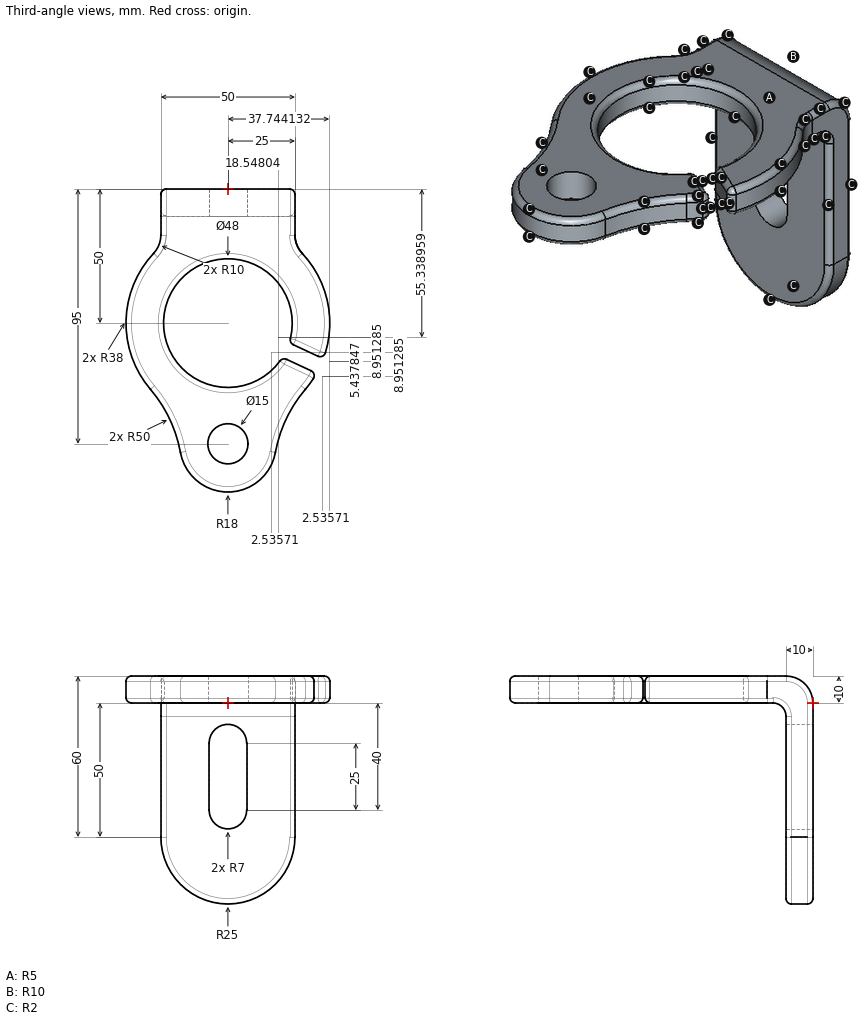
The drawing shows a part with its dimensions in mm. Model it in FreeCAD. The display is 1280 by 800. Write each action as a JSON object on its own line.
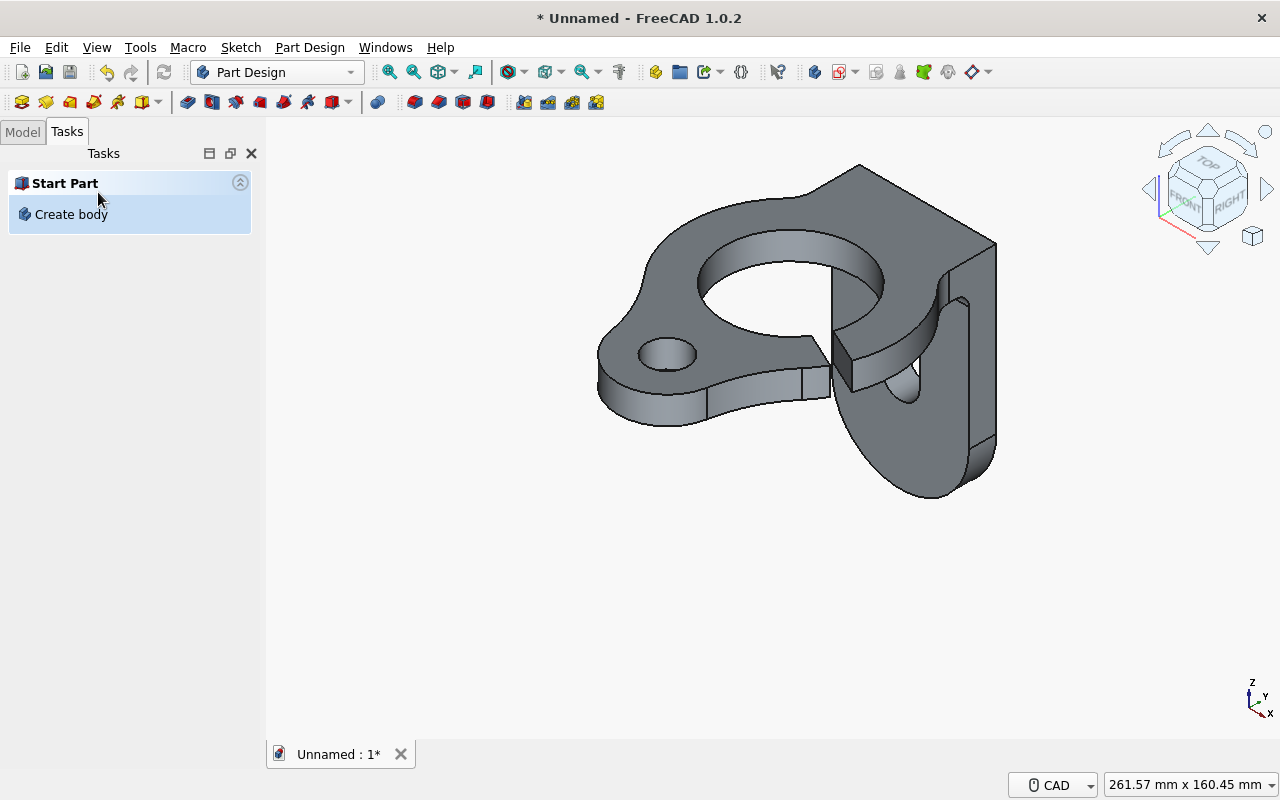
{"action": "key", "text": "2"}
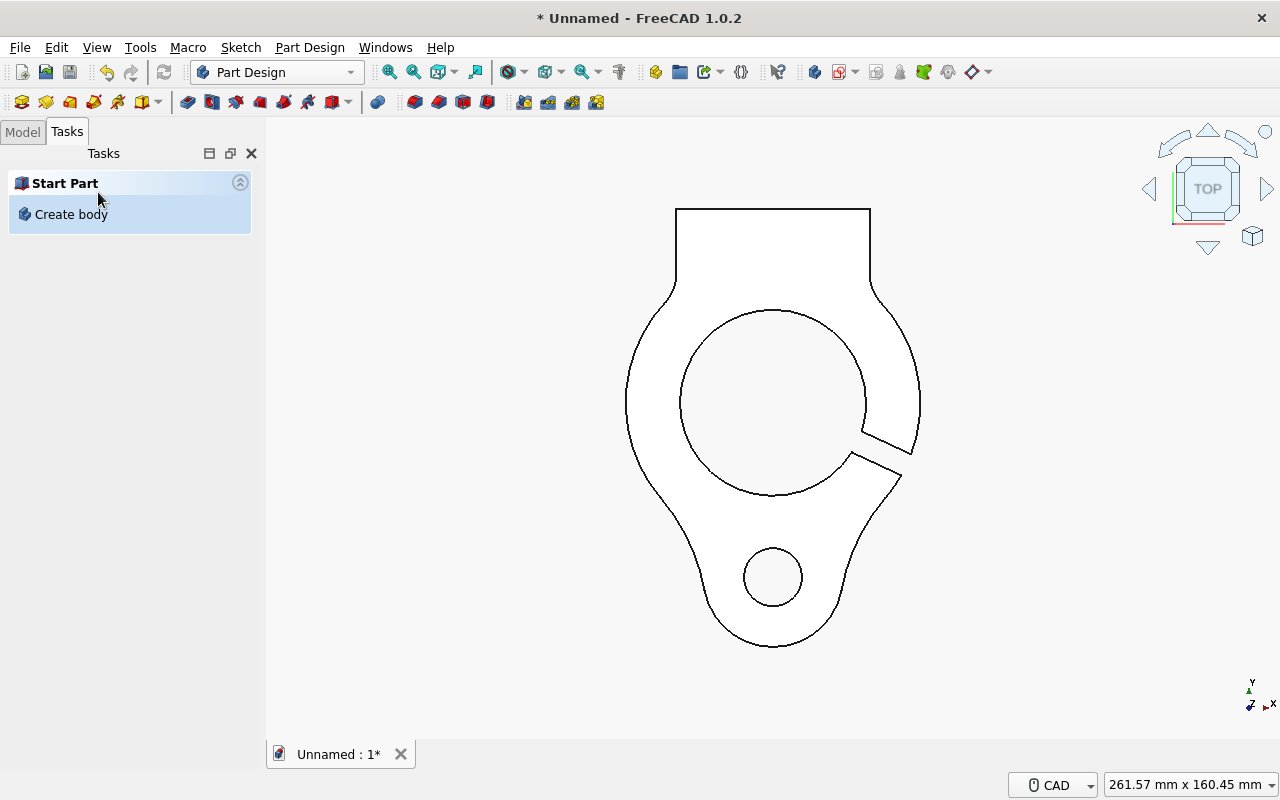
{"action": "left_click", "coordinate": [773, 208]}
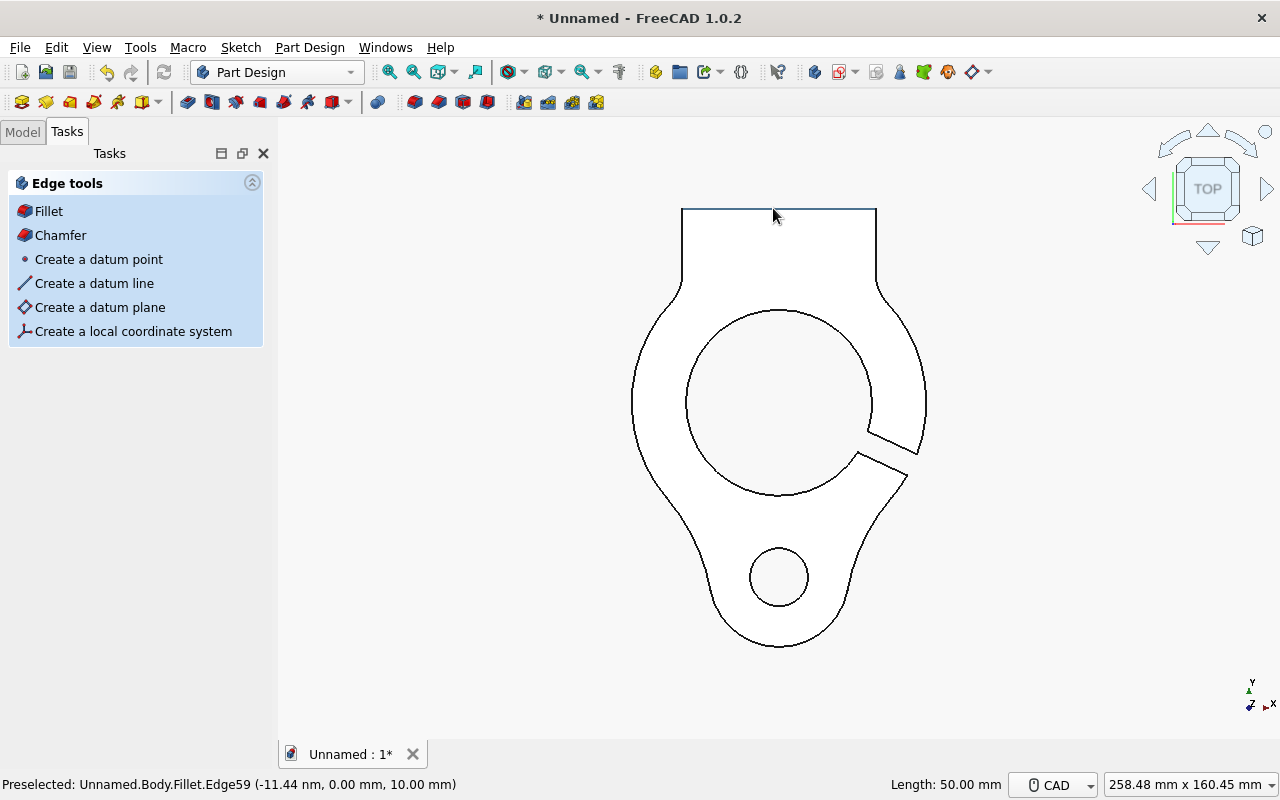
{"action": "left_click", "coordinate": [416, 102]}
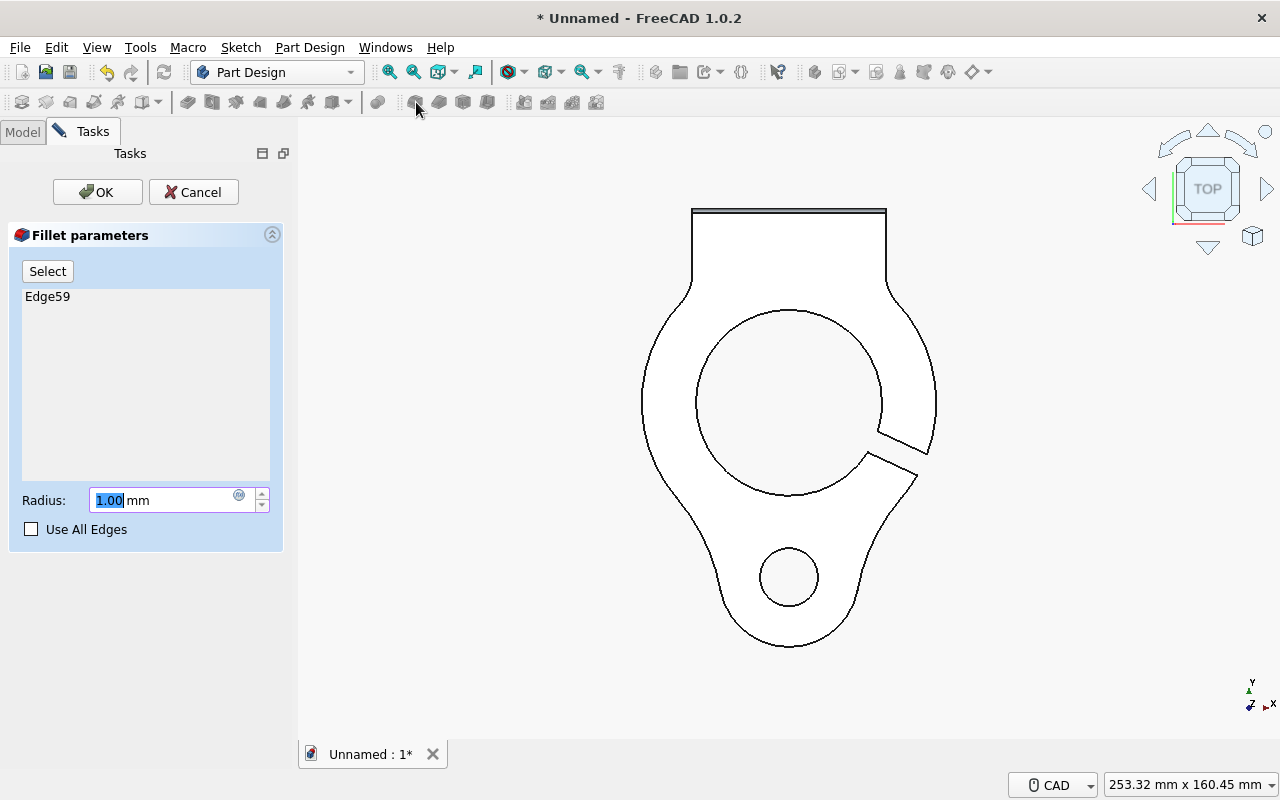
{"action": "type", "text": "10"}
{"action": "key", "text": "Tab"}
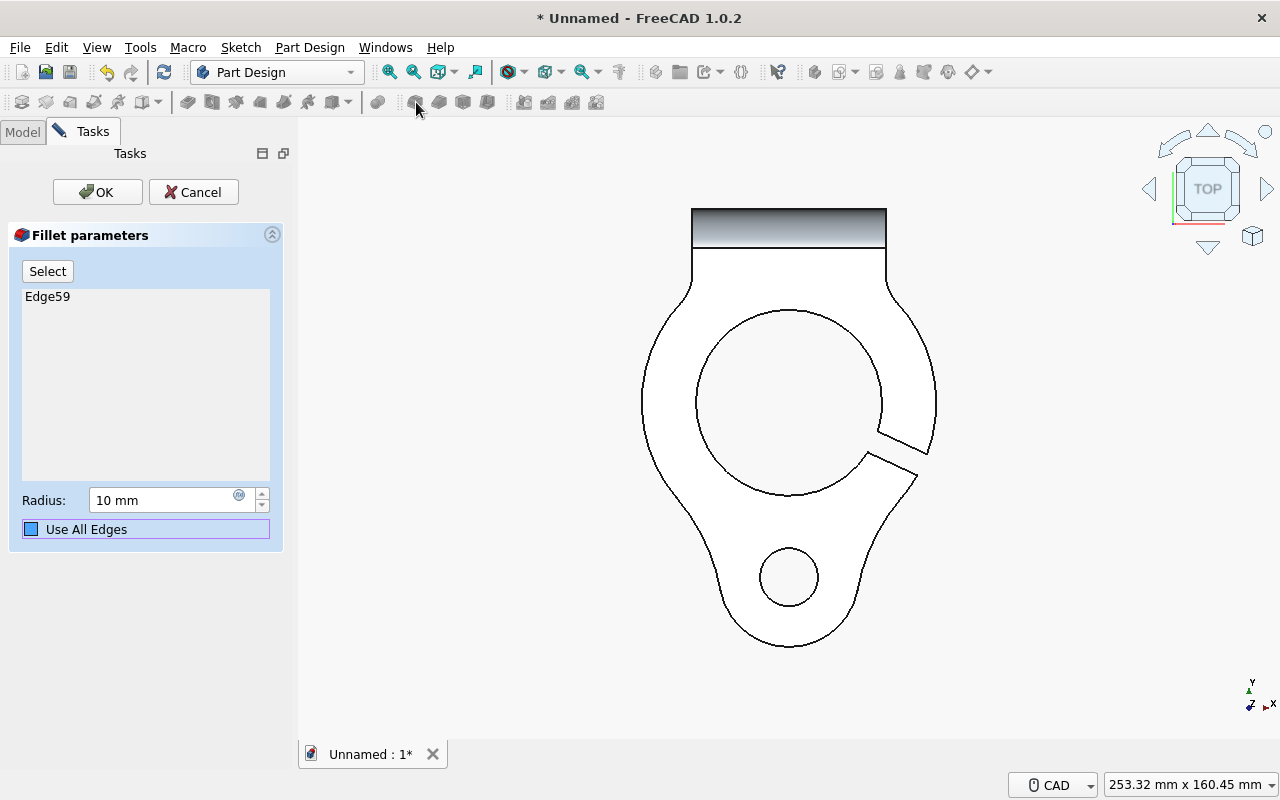
{"action": "left_click", "coordinate": [98, 192]}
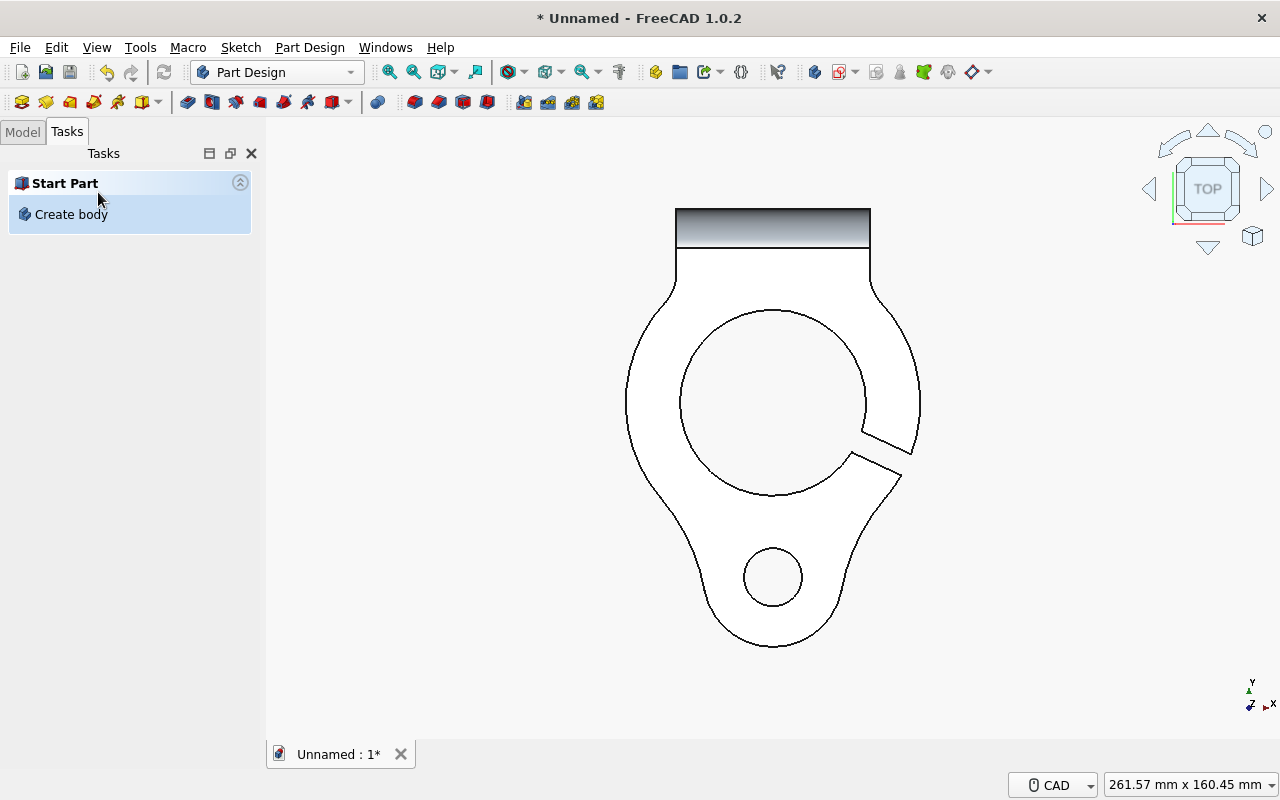
{"action": "left_click", "coordinate": [676, 261]}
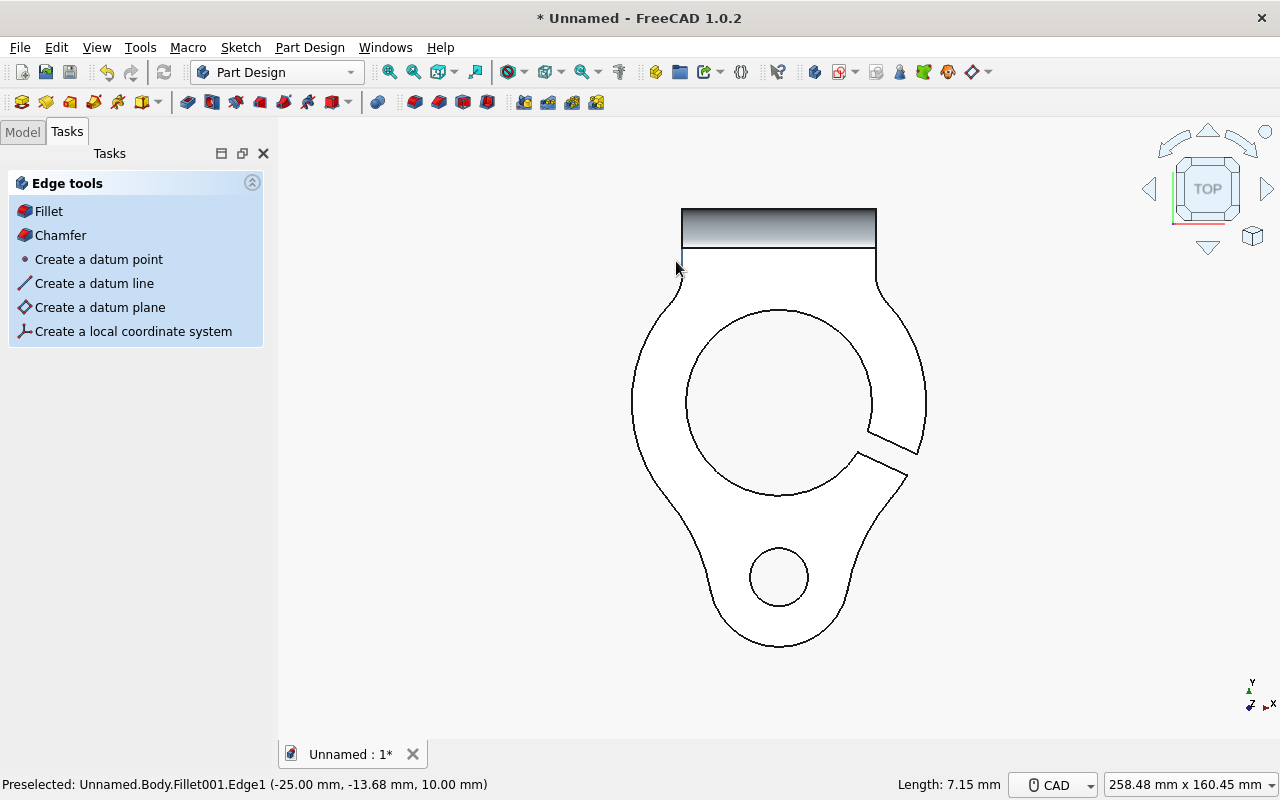
{"action": "left_click", "coordinate": [682, 219], "text": "ctrl"}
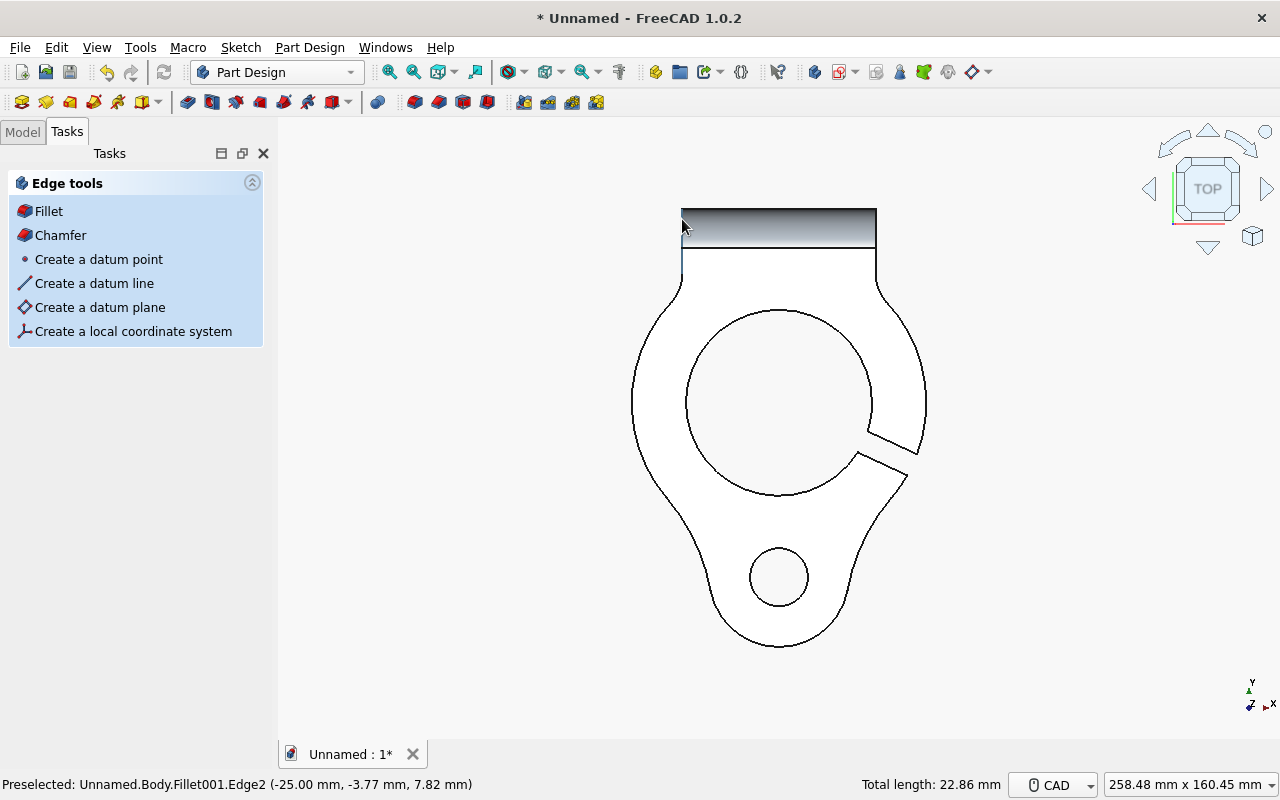
{"action": "left_click", "coordinate": [876, 219], "text": "ctrl"}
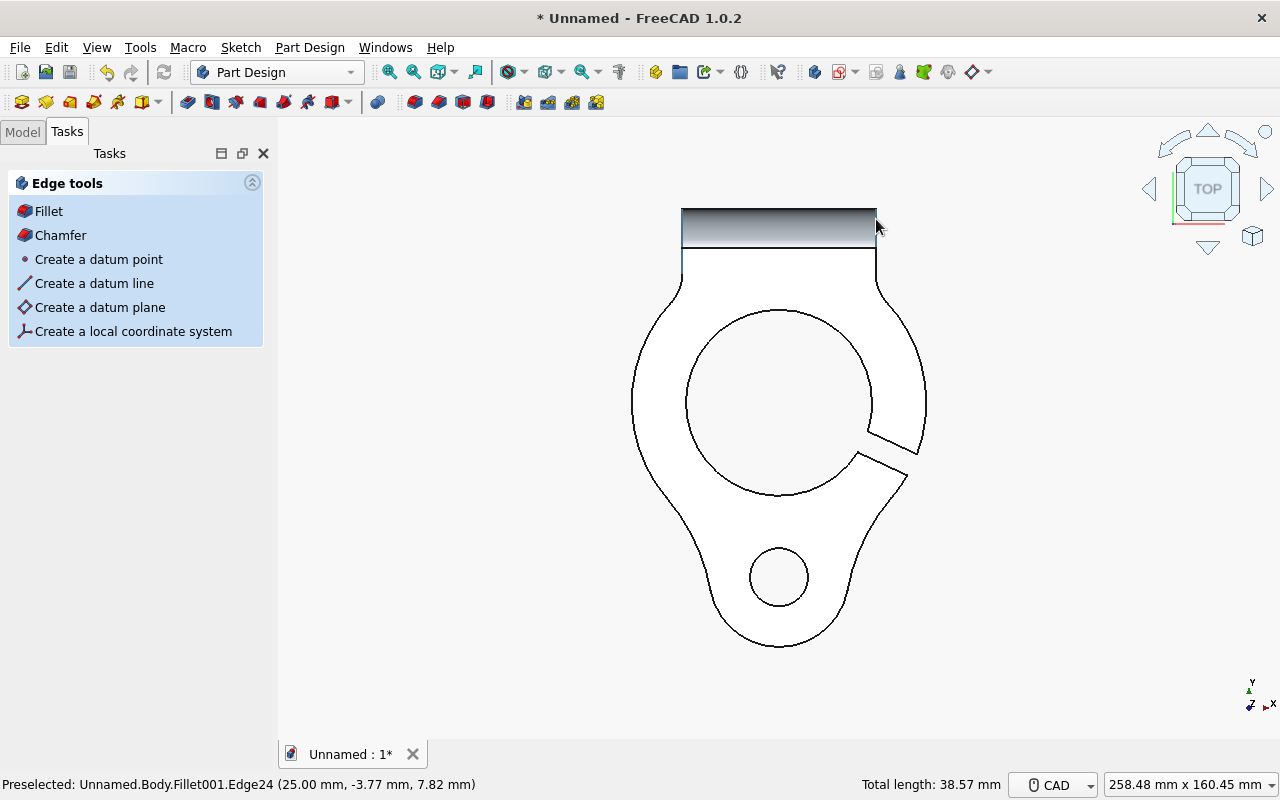
{"action": "left_click", "coordinate": [863, 540], "text": "ctrl"}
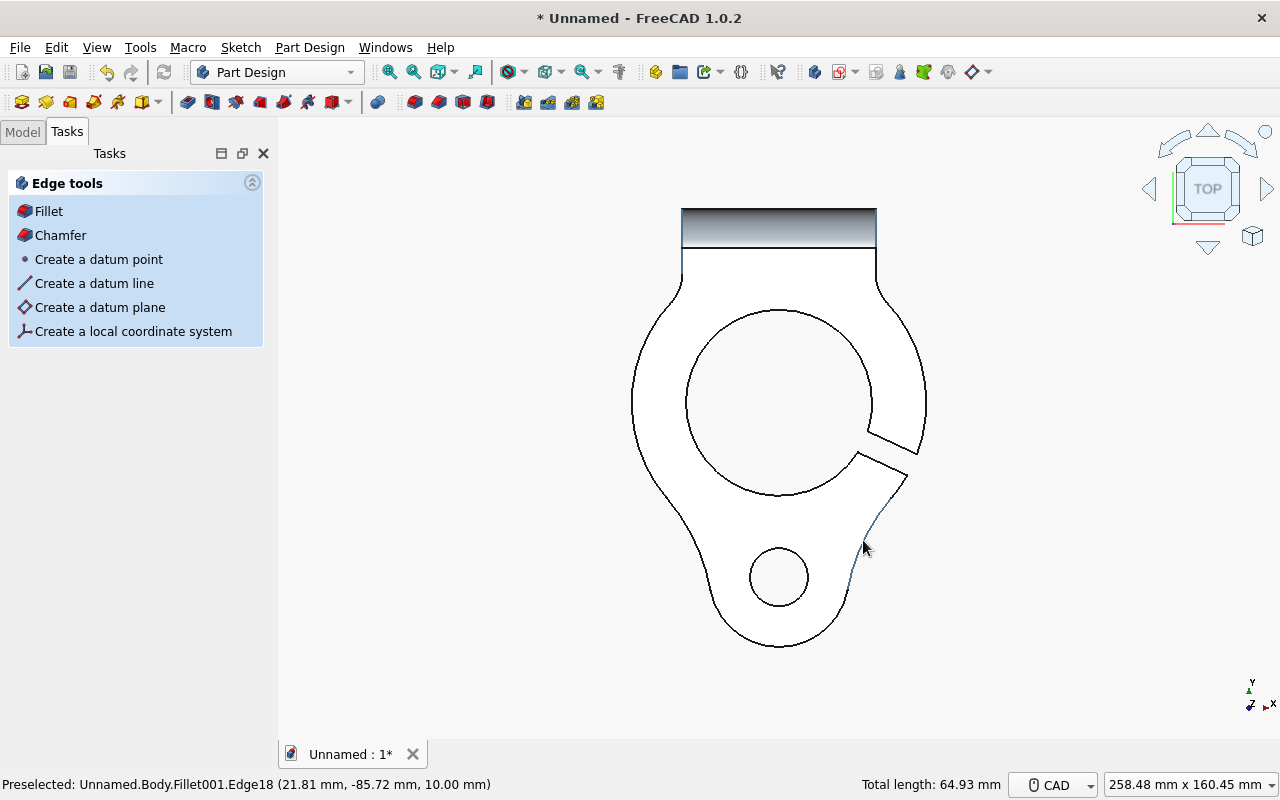
{"action": "left_click", "coordinate": [900, 486], "text": "ctrl"}